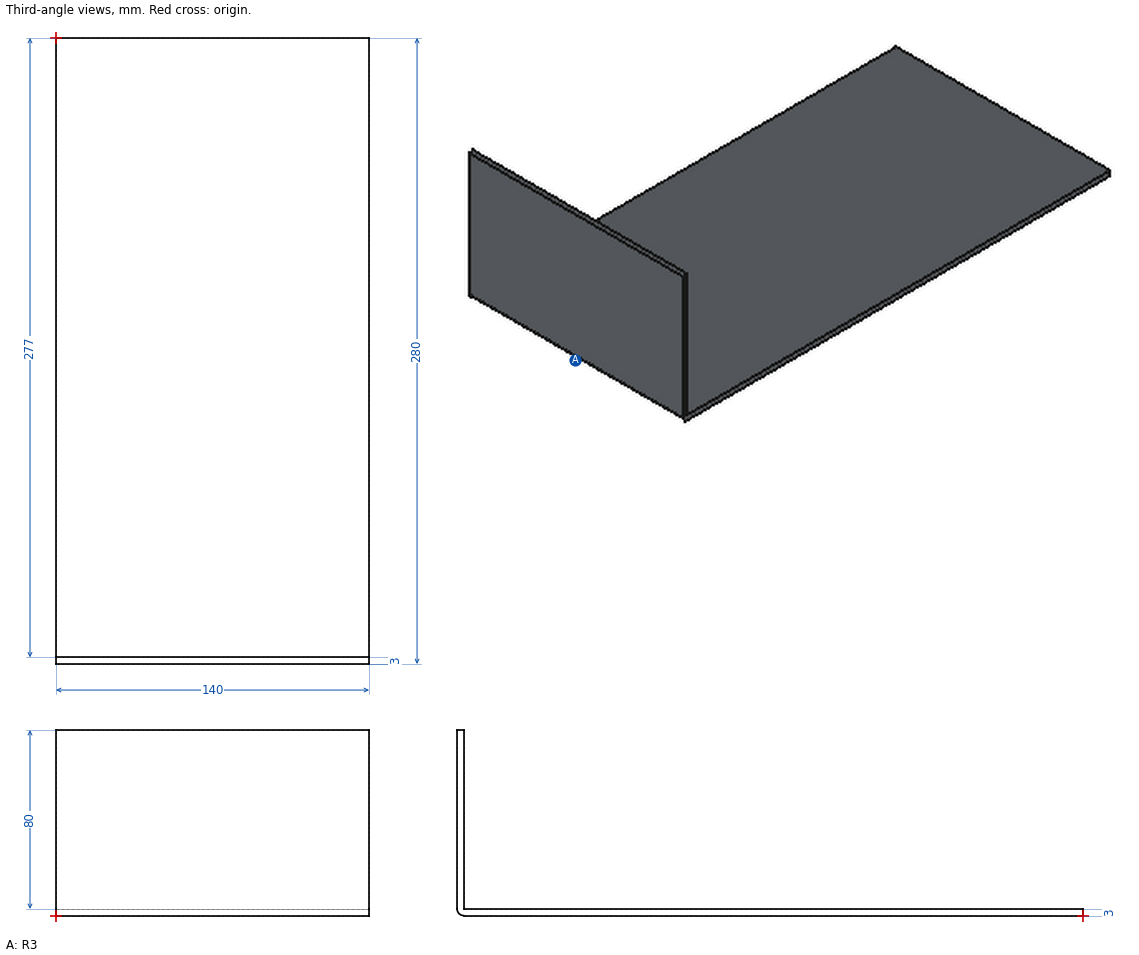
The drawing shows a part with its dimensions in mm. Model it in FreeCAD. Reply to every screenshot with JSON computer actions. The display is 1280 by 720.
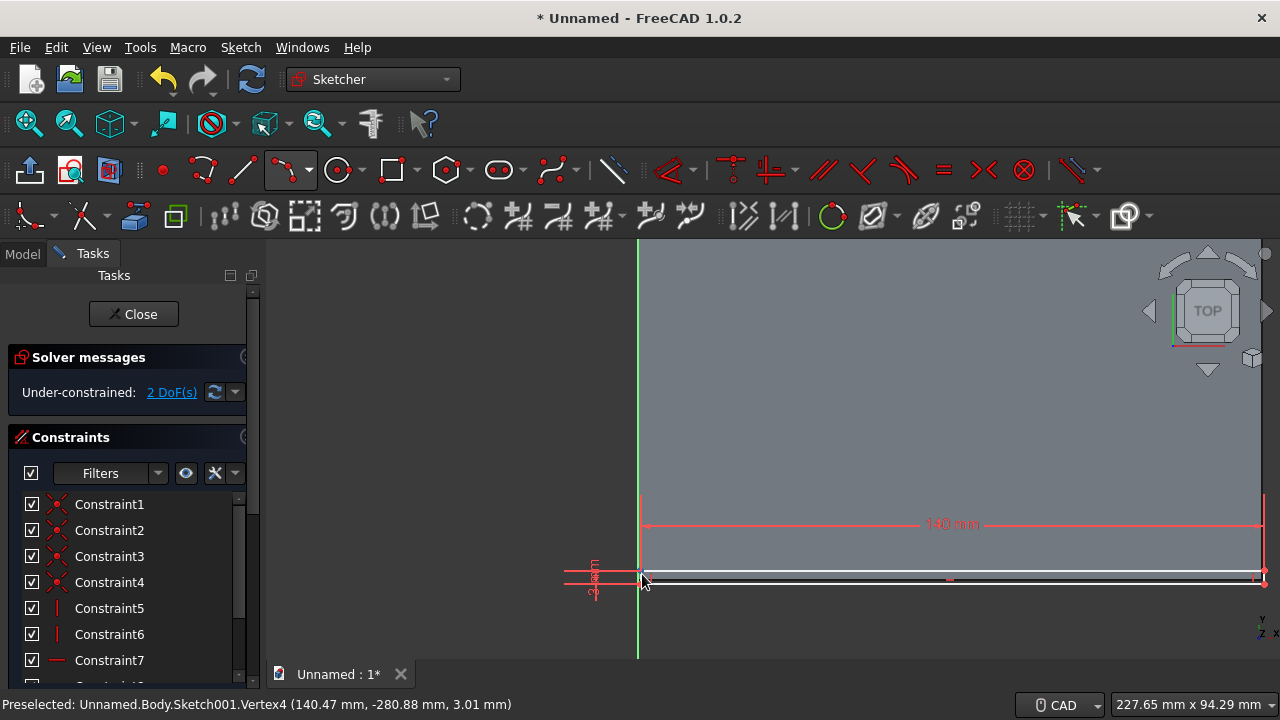
{"action": "left_click", "coordinate": [641, 571]}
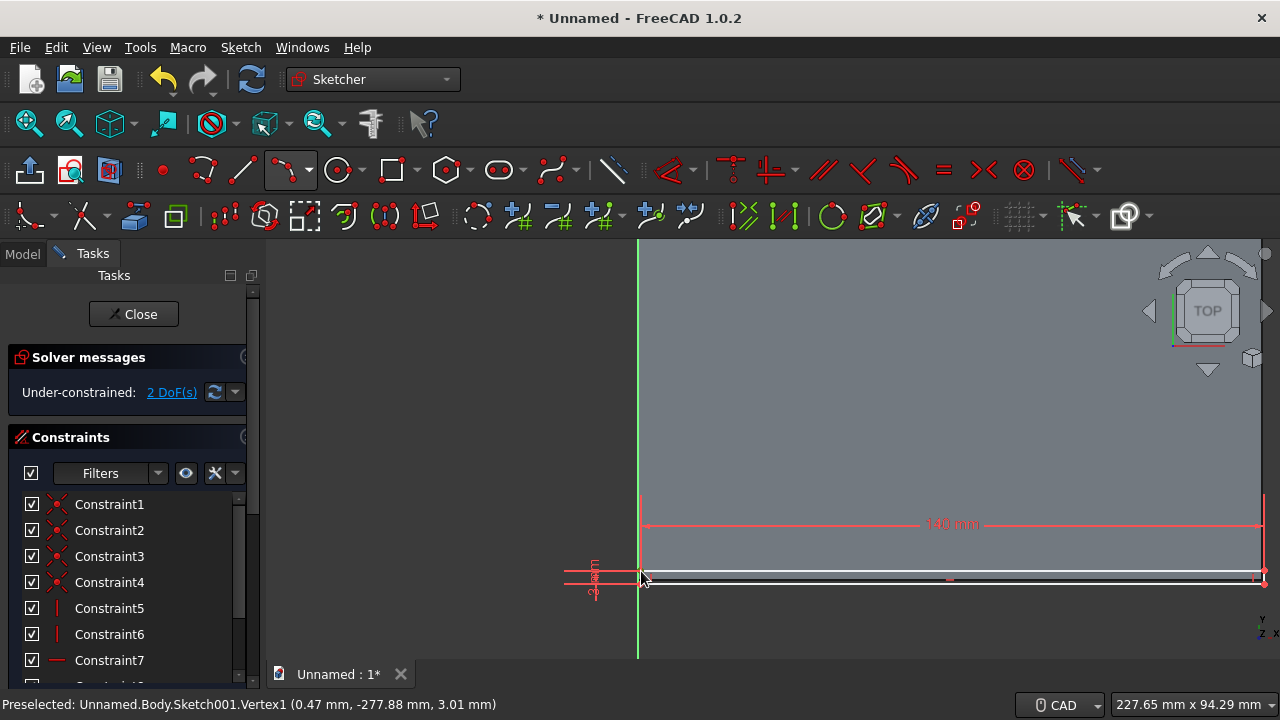
{"action": "left_click", "coordinate": [638, 527]}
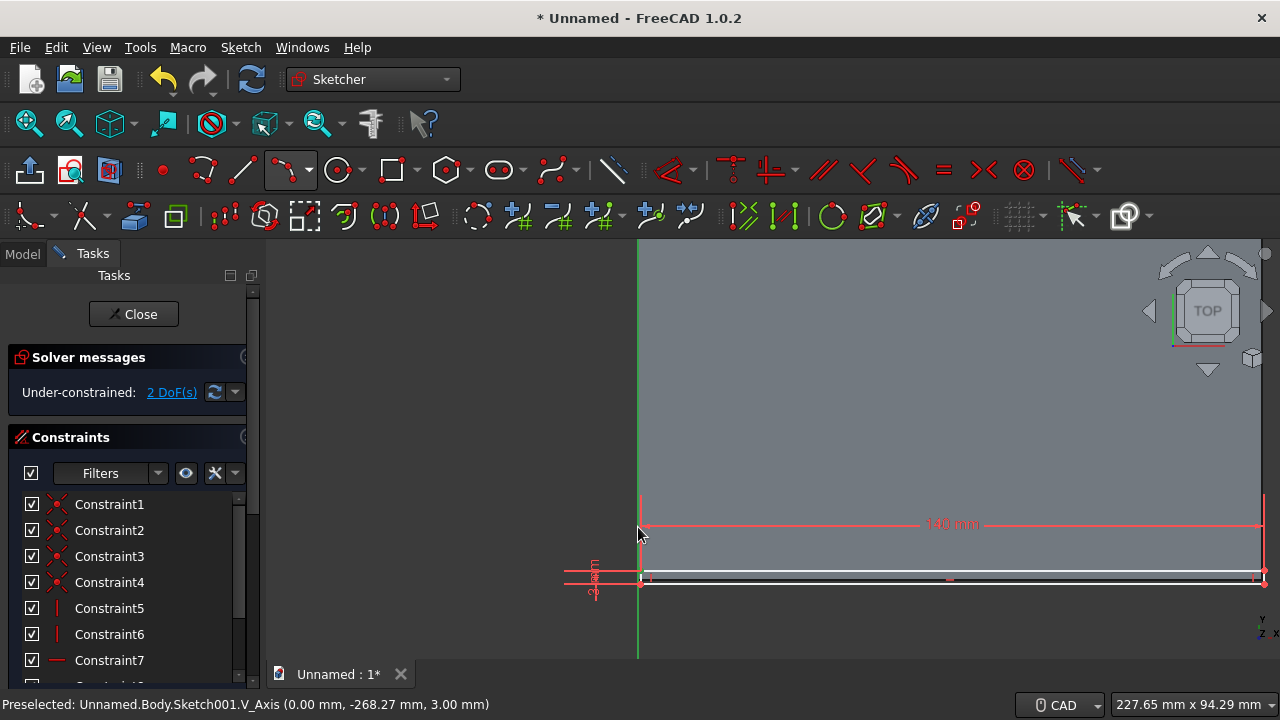
{"action": "left_click", "coordinate": [732, 170]}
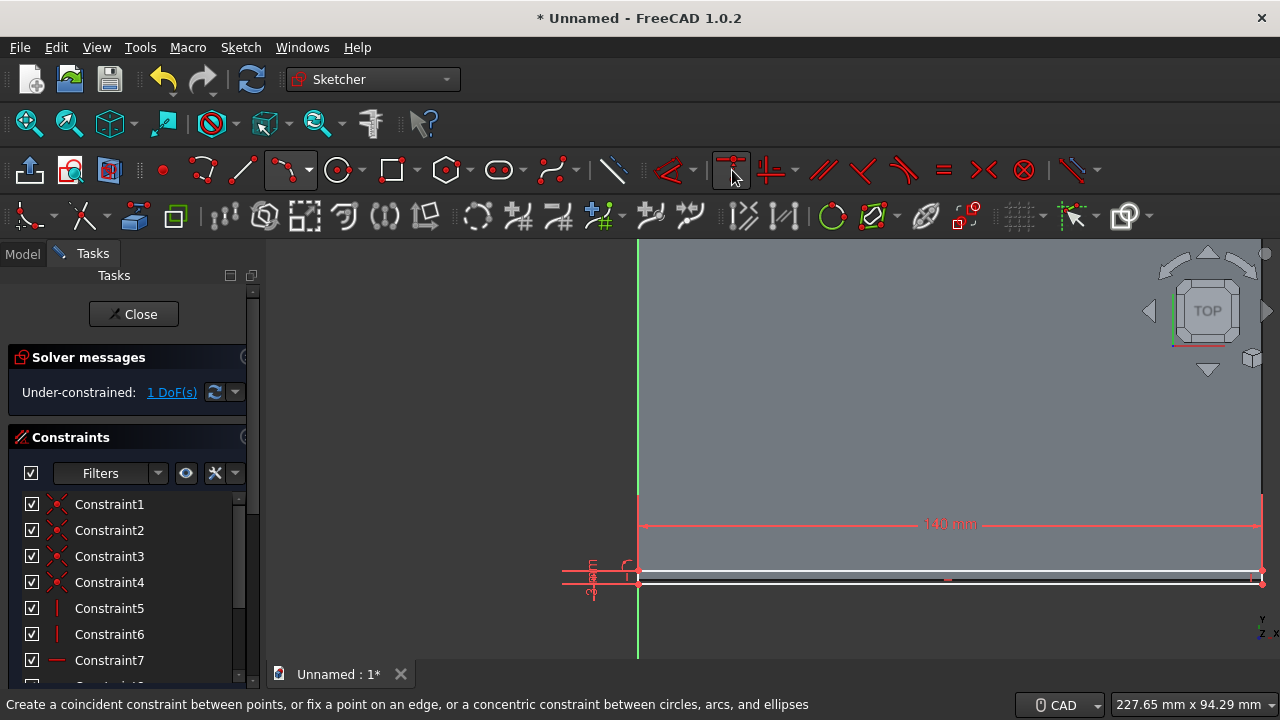
{"action": "left_click", "coordinate": [638, 571]}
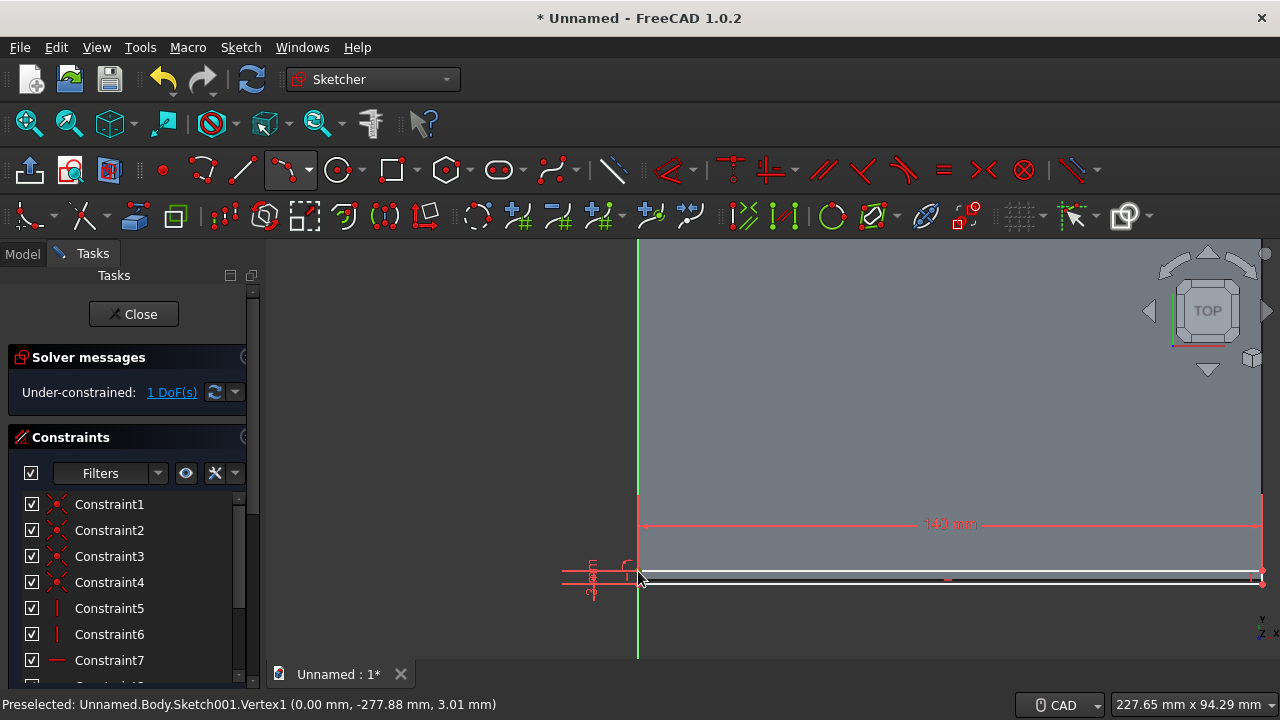
{"action": "key", "text": "i"}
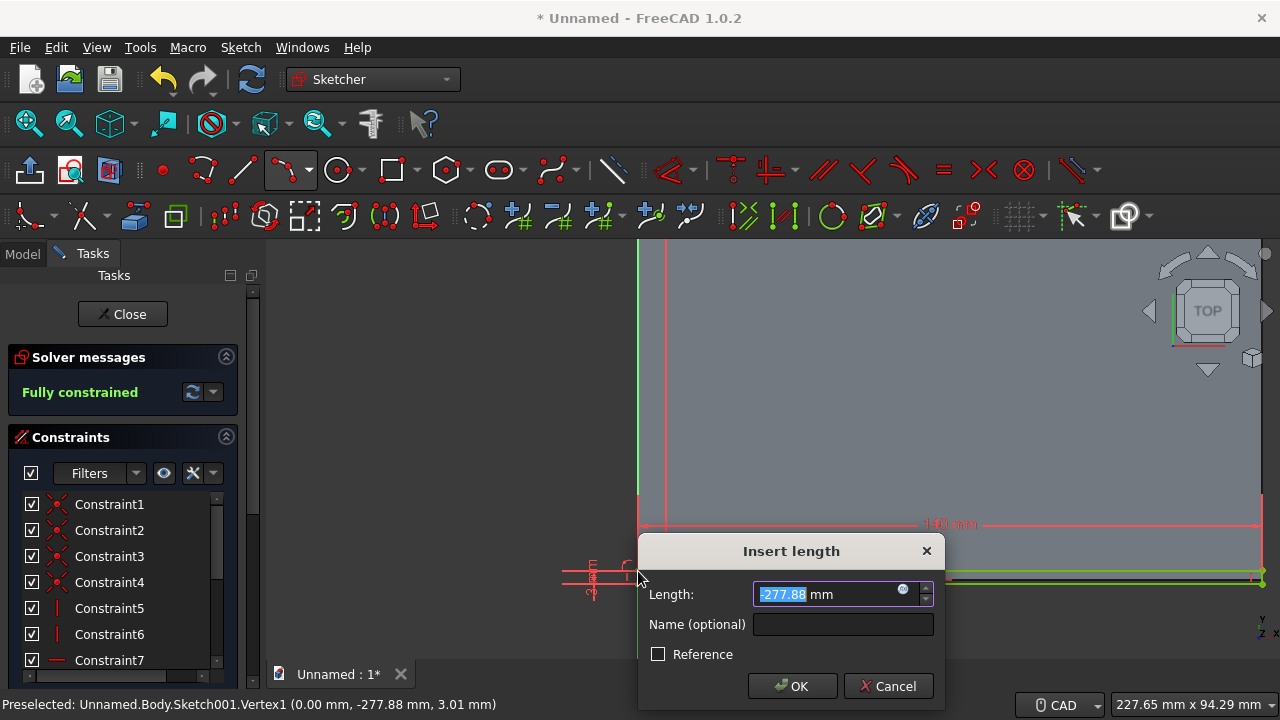
{"action": "type", "text": "-277"}
{"action": "key", "text": "Return"}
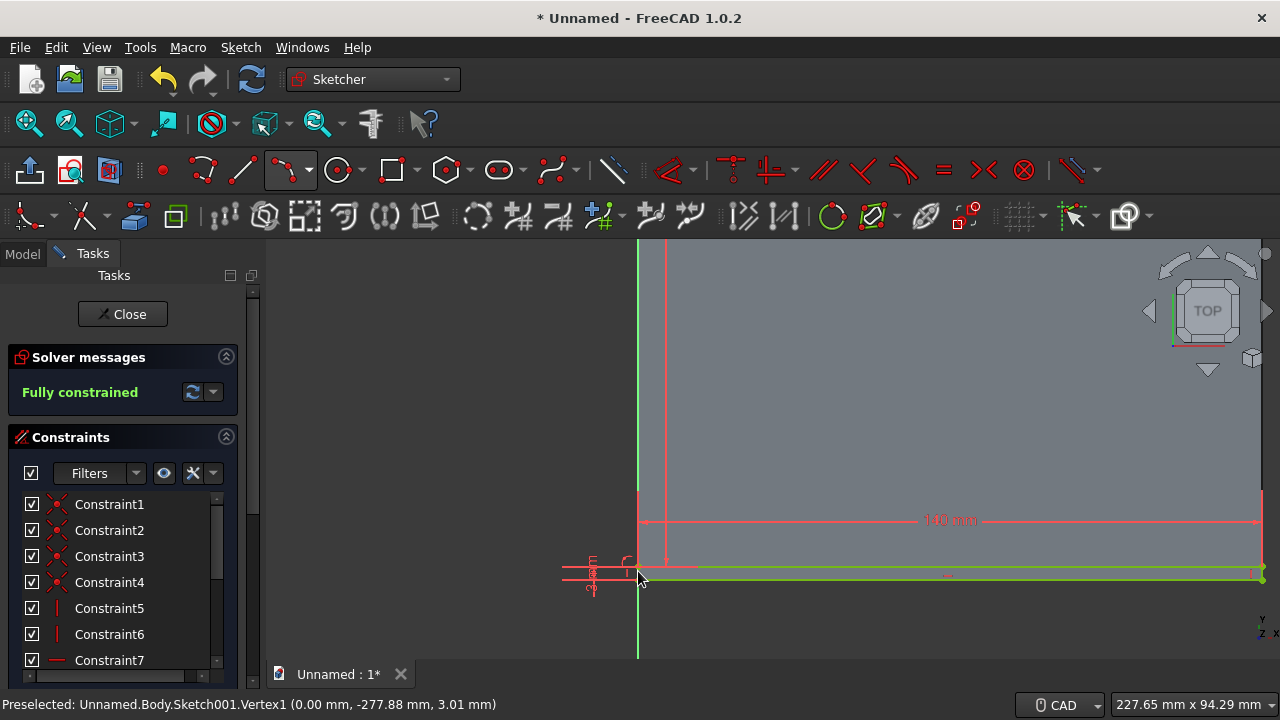
{"action": "left_click", "coordinate": [123, 314]}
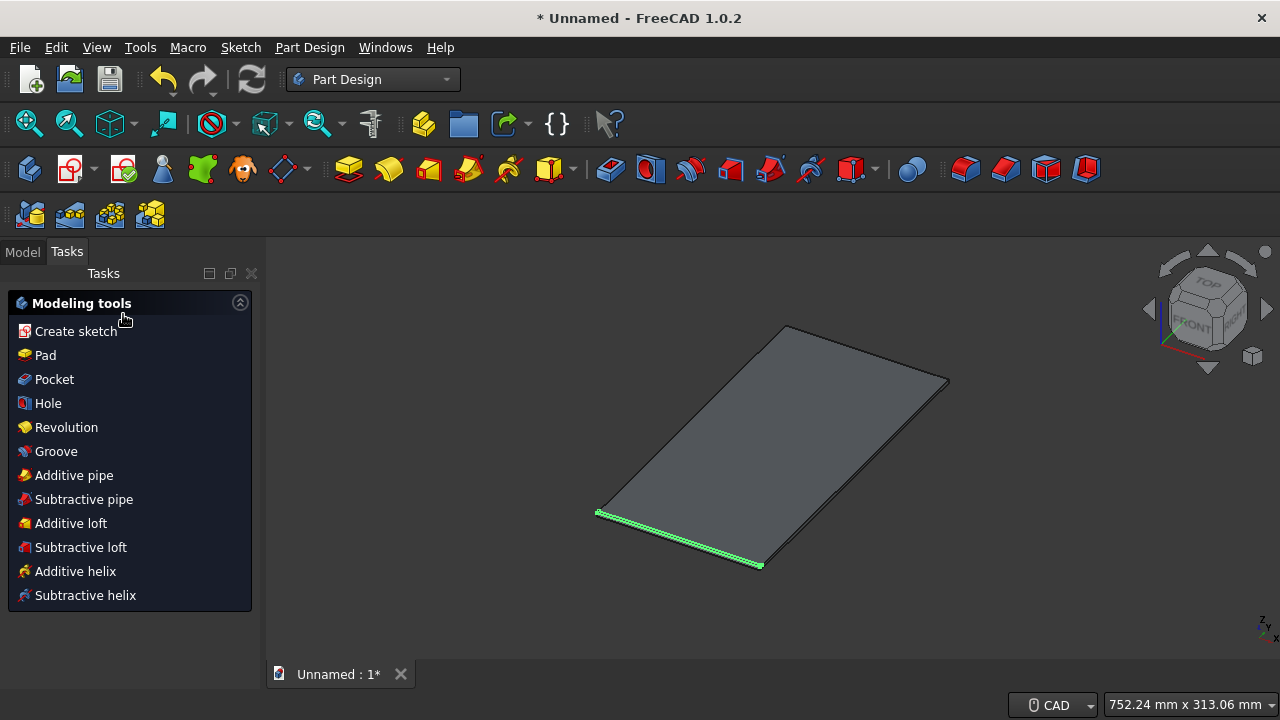
{"action": "left_click", "coordinate": [350, 170]}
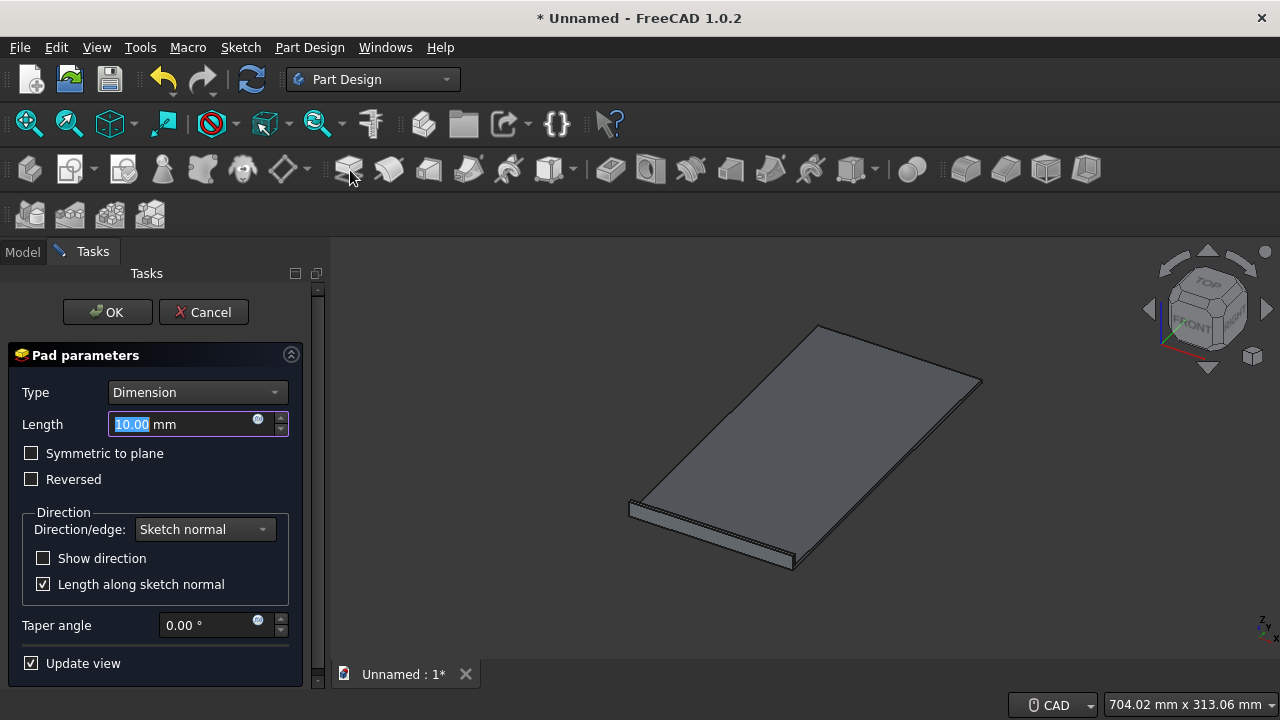
{"action": "type", "text": "80"}
{"action": "key", "text": "Tab"}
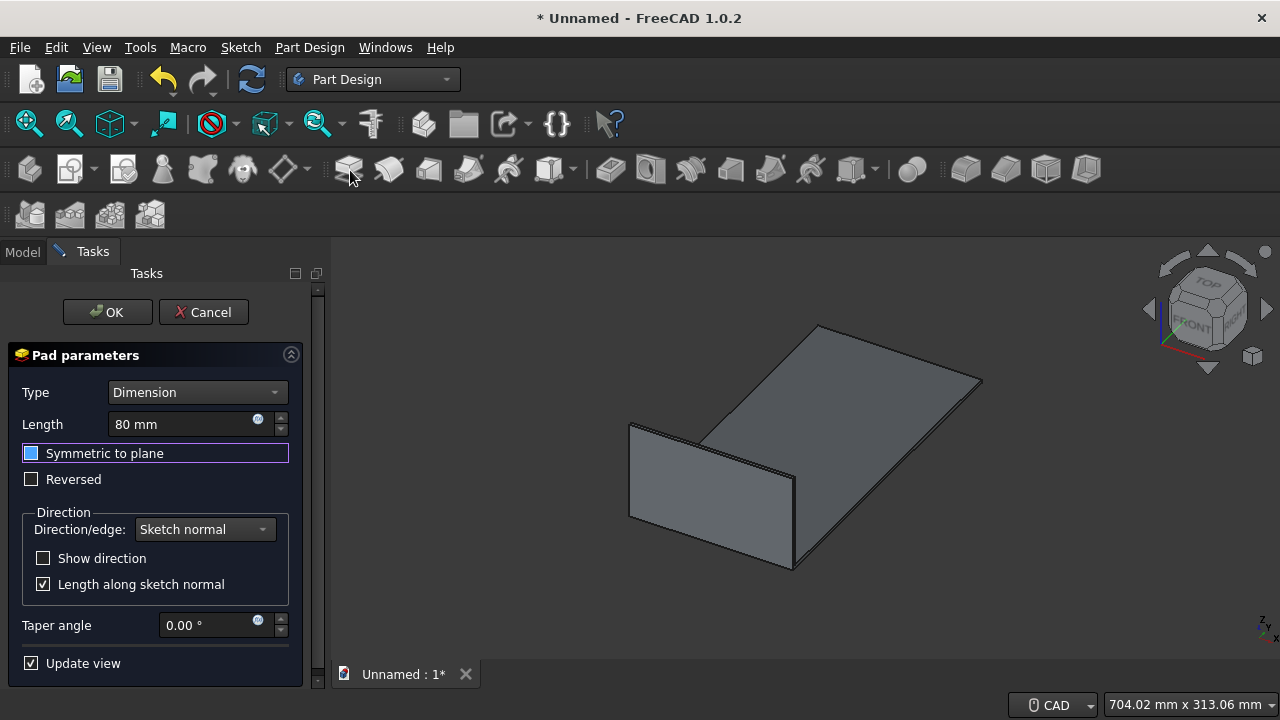
{"action": "left_click", "coordinate": [108, 312]}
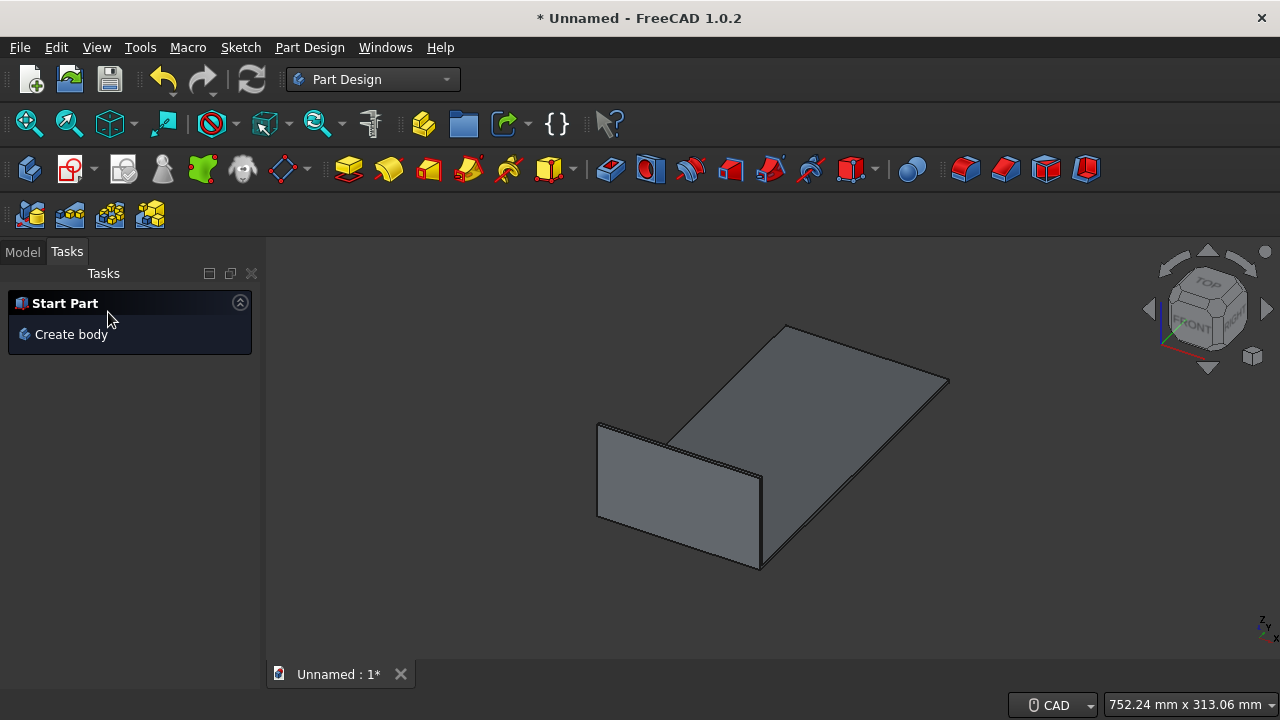
{"action": "key", "text": "v f"}